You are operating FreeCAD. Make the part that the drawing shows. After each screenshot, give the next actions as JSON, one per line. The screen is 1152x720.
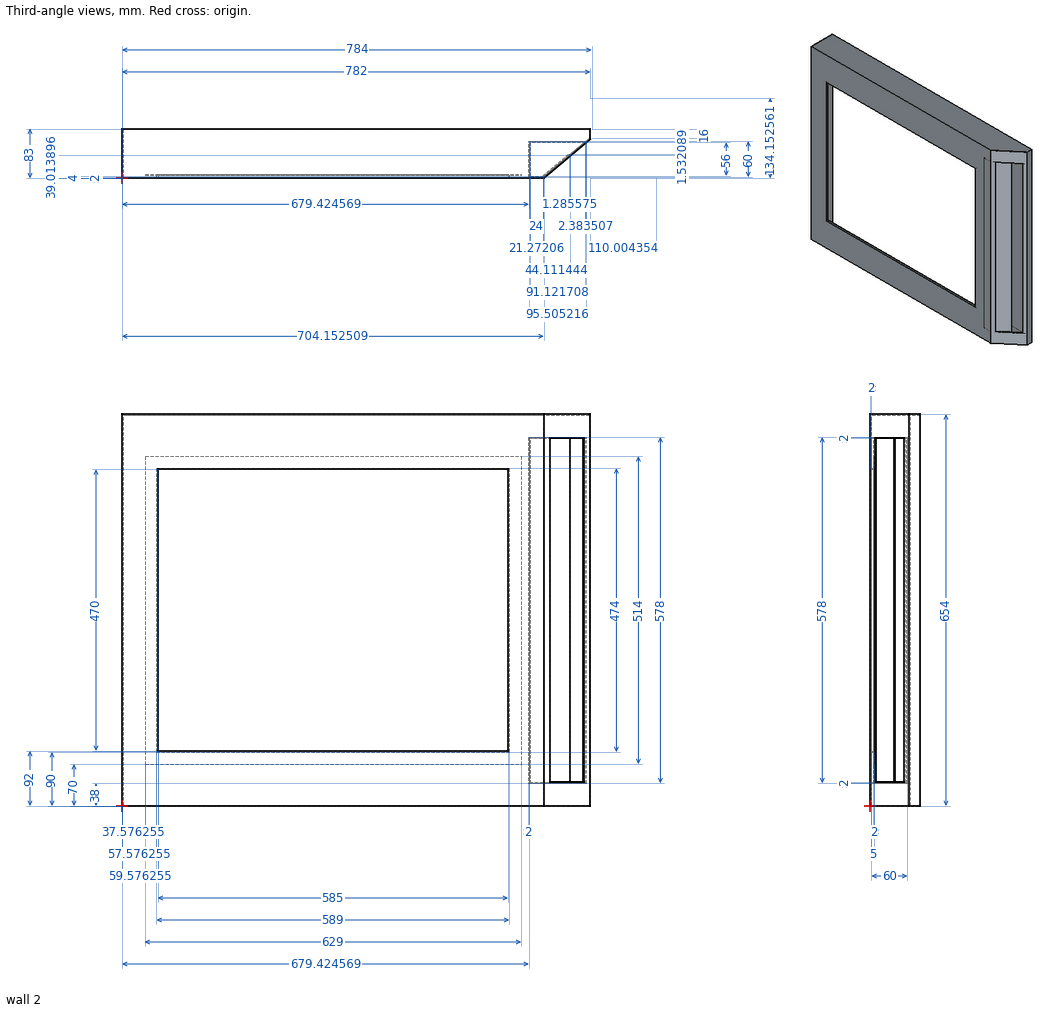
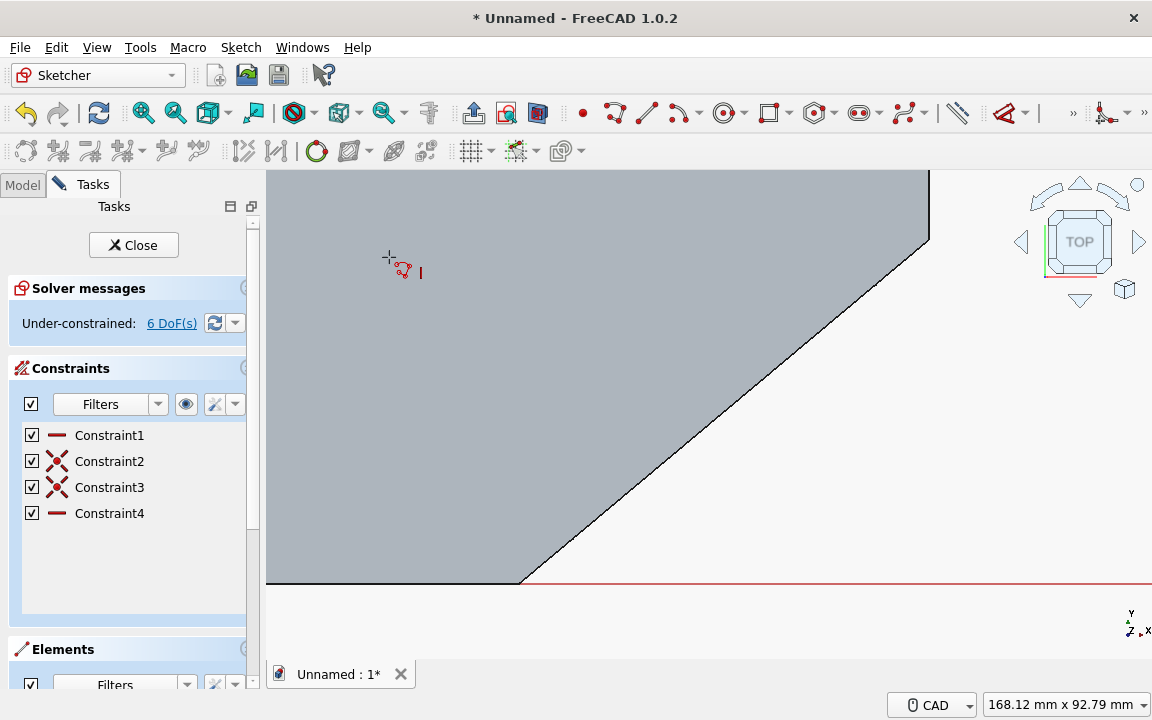
{"action": "scroll", "coordinate": [389, 573], "scroll_direction": "up", "scroll_amount": 3}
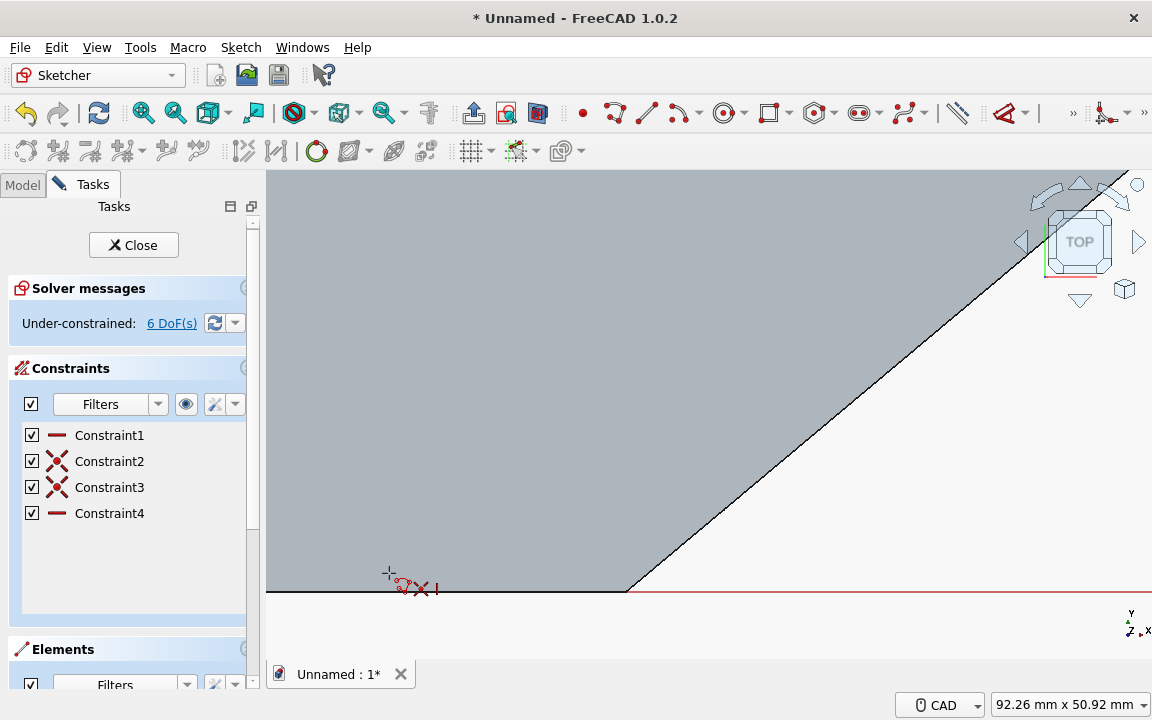
{"action": "left_click", "coordinate": [388, 573]}
{"action": "key", "text": "Escape"}
{"action": "key", "text": "Escape"}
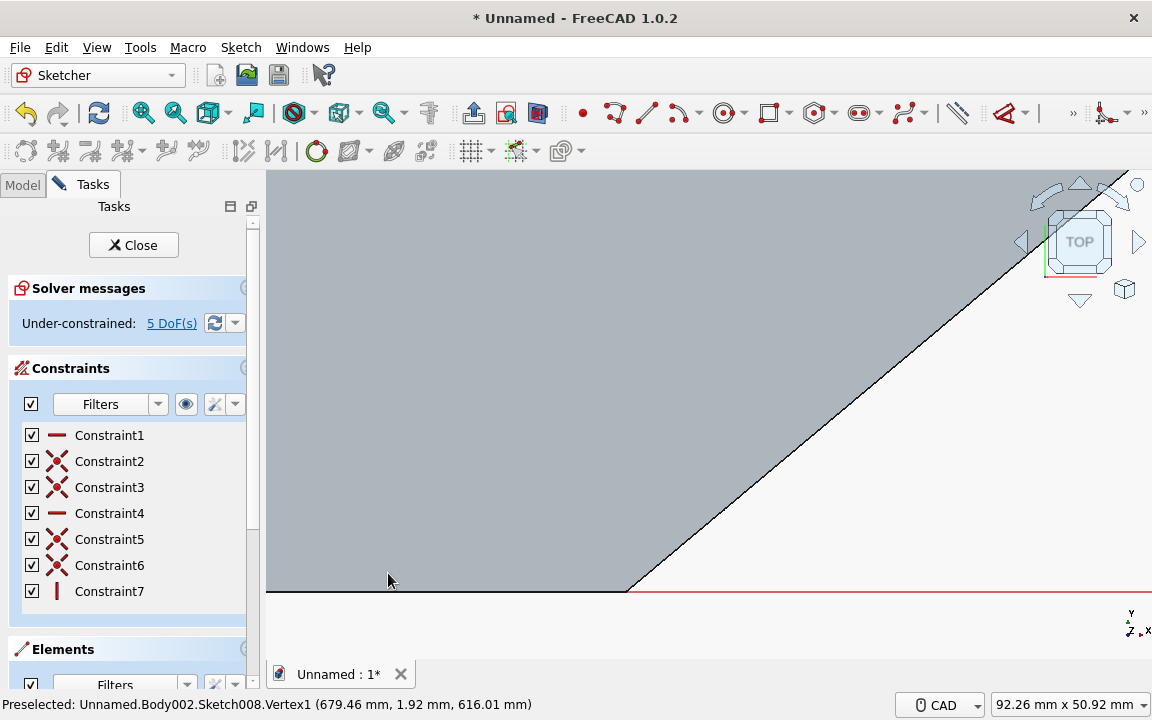
{"action": "key", "text": "d"}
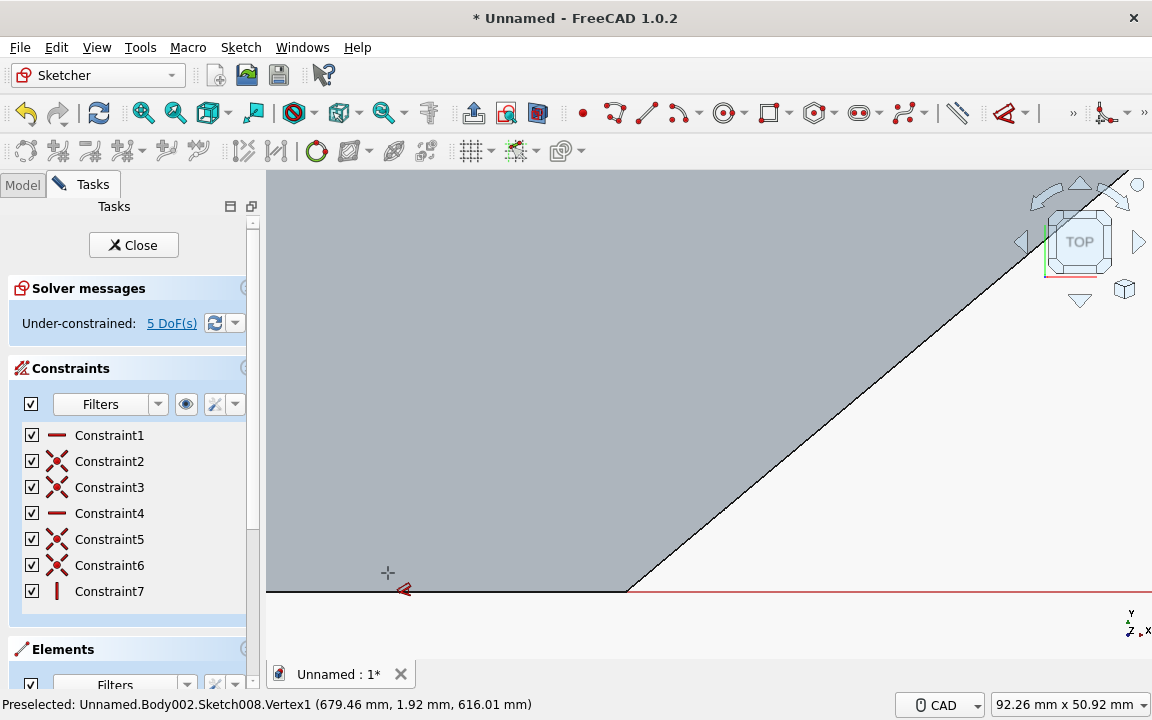
{"action": "left_click", "coordinate": [458, 573]}
{"action": "left_click", "coordinate": [504, 607]}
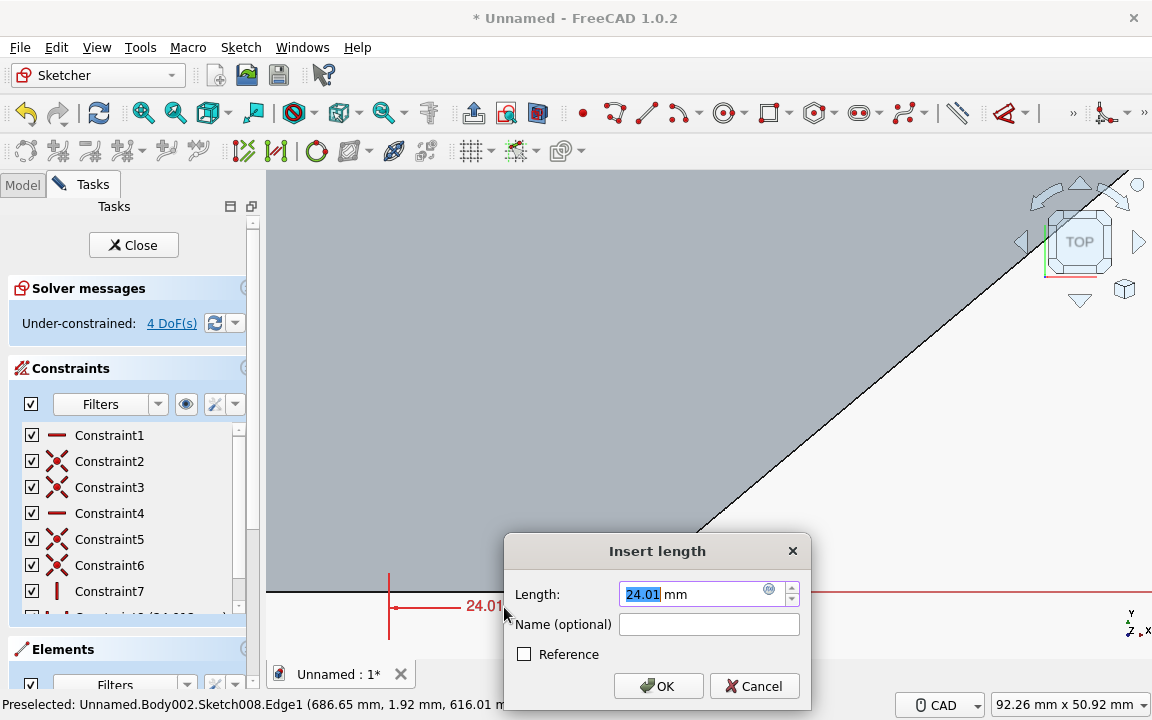
{"action": "type", "text": "24"}
{"action": "key", "text": "Return"}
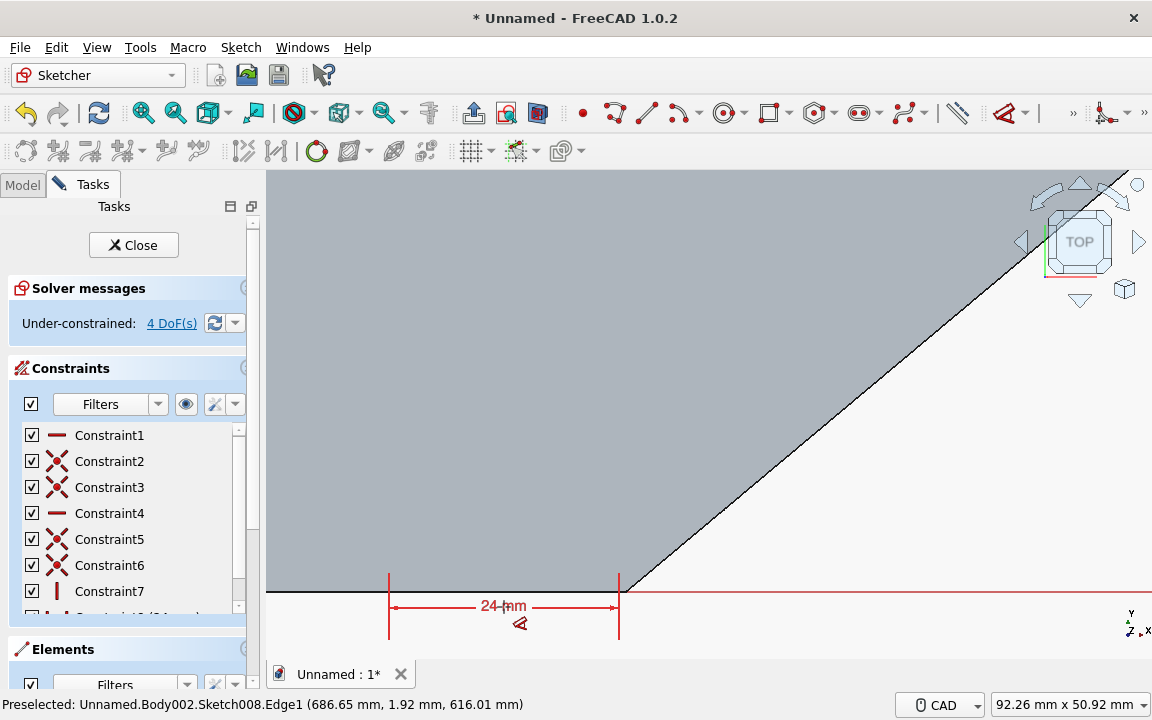
{"action": "left_click", "coordinate": [389, 401]}
{"action": "left_click", "coordinate": [355, 386]}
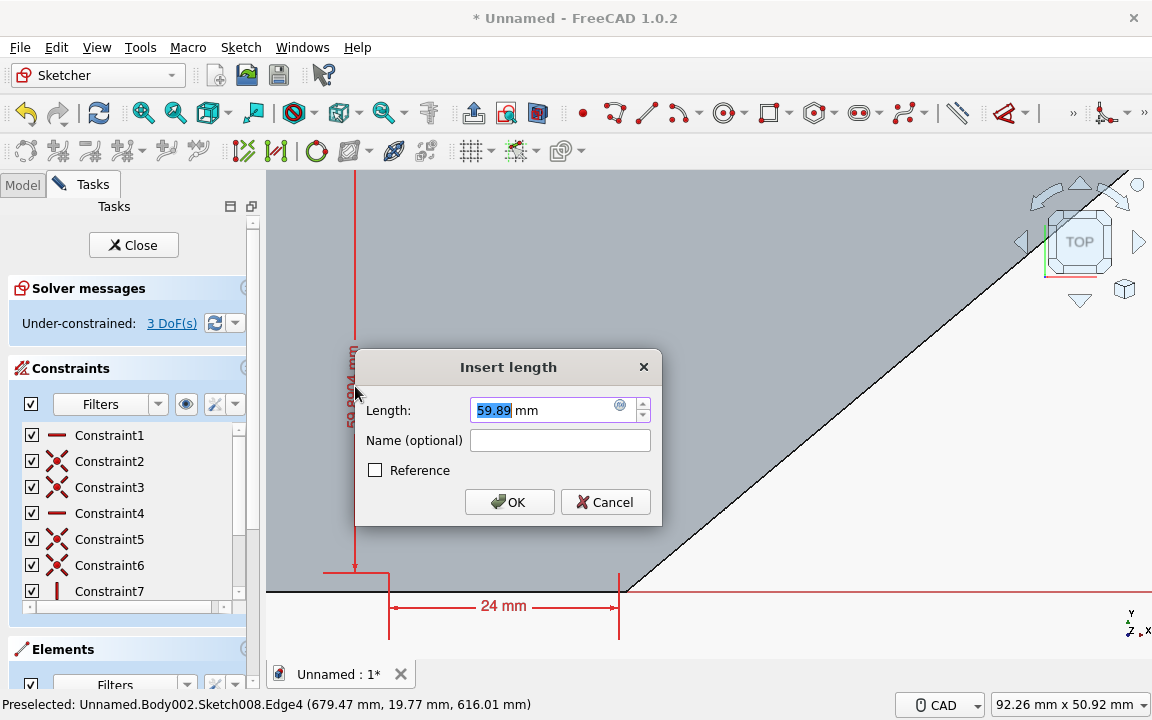
{"action": "type", "text": "60"}
{"action": "key", "text": "Return"}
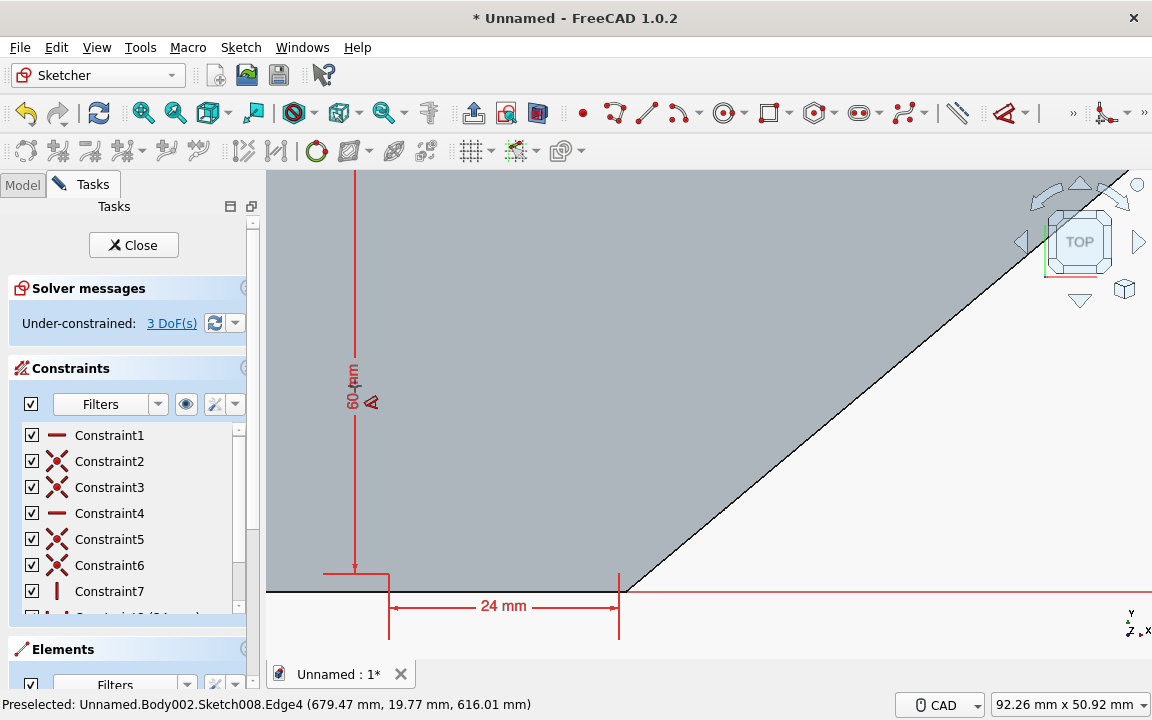
{"action": "scroll", "coordinate": [389, 574], "scroll_direction": "up", "scroll_amount": 4}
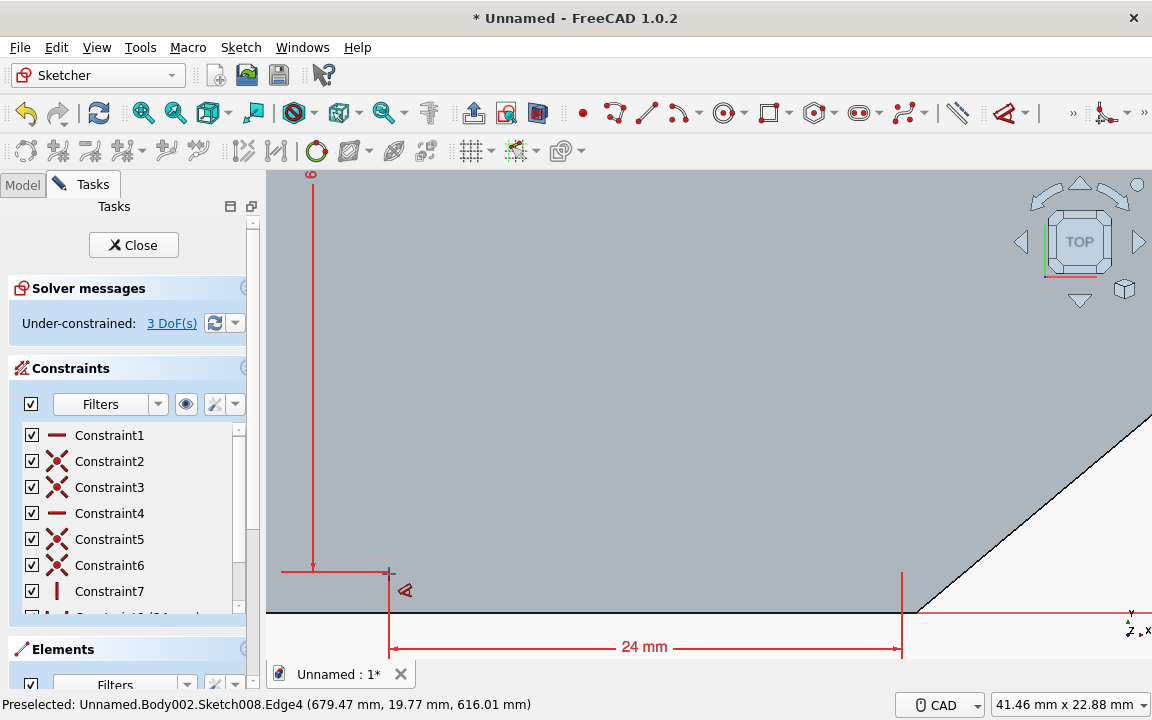
{"action": "left_click", "coordinate": [389, 572]}
{"action": "left_click", "coordinate": [423, 592]}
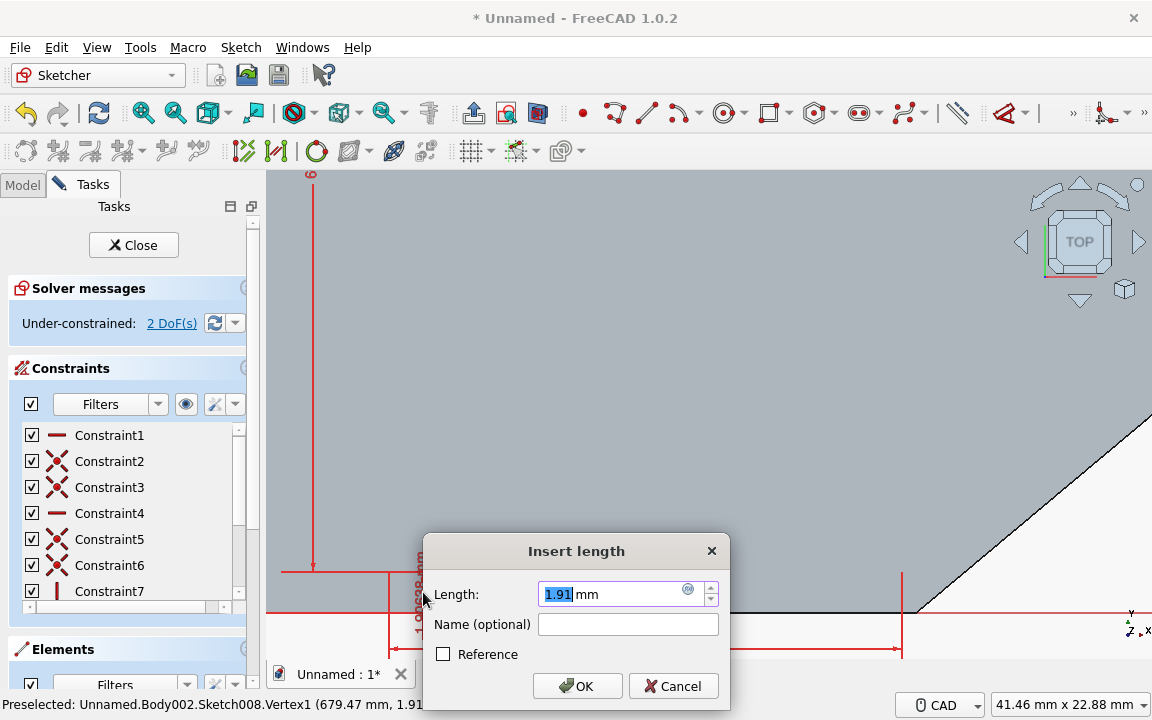
{"action": "type", "text": "2"}
{"action": "key", "text": "Return"}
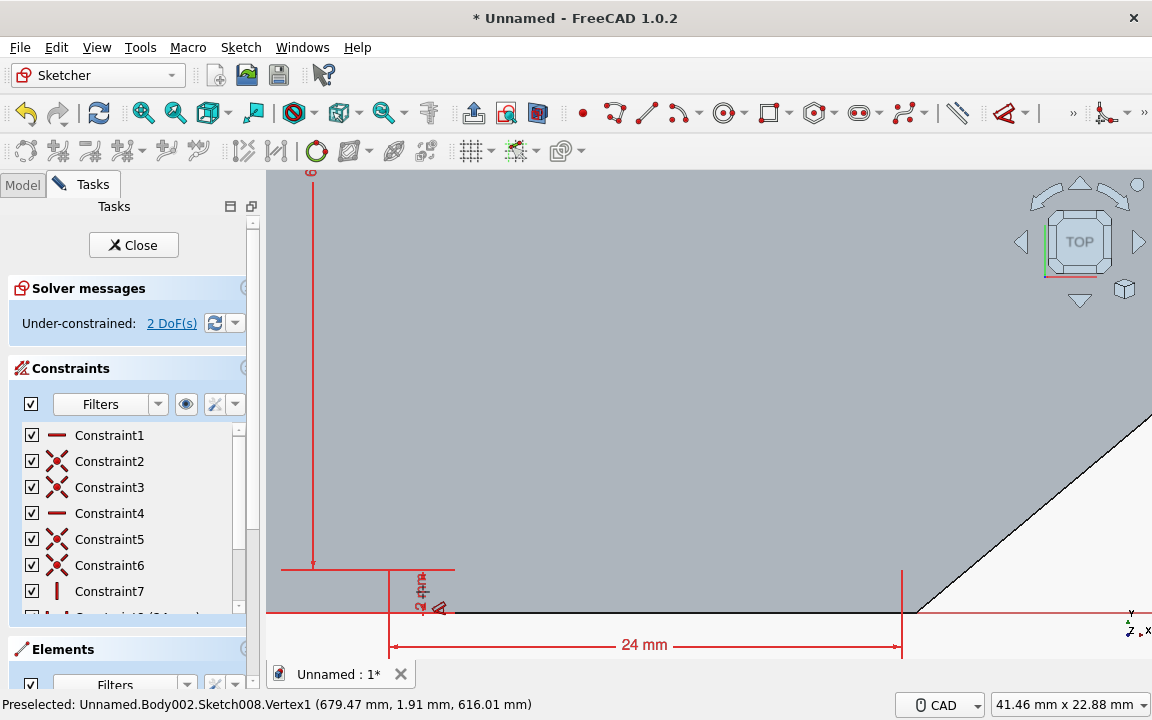
{"action": "scroll", "coordinate": [389, 573], "scroll_direction": "down", "scroll_amount": 7}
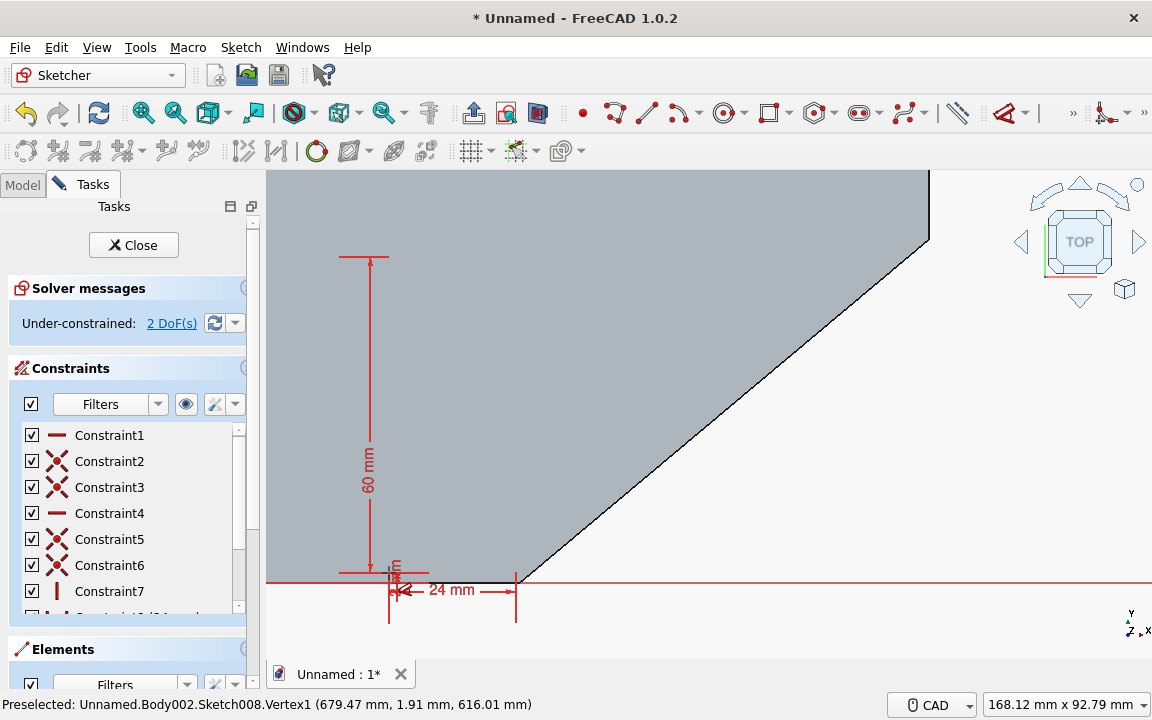
{"action": "left_click", "coordinate": [741, 257]}
{"action": "left_click", "coordinate": [641, 223]}